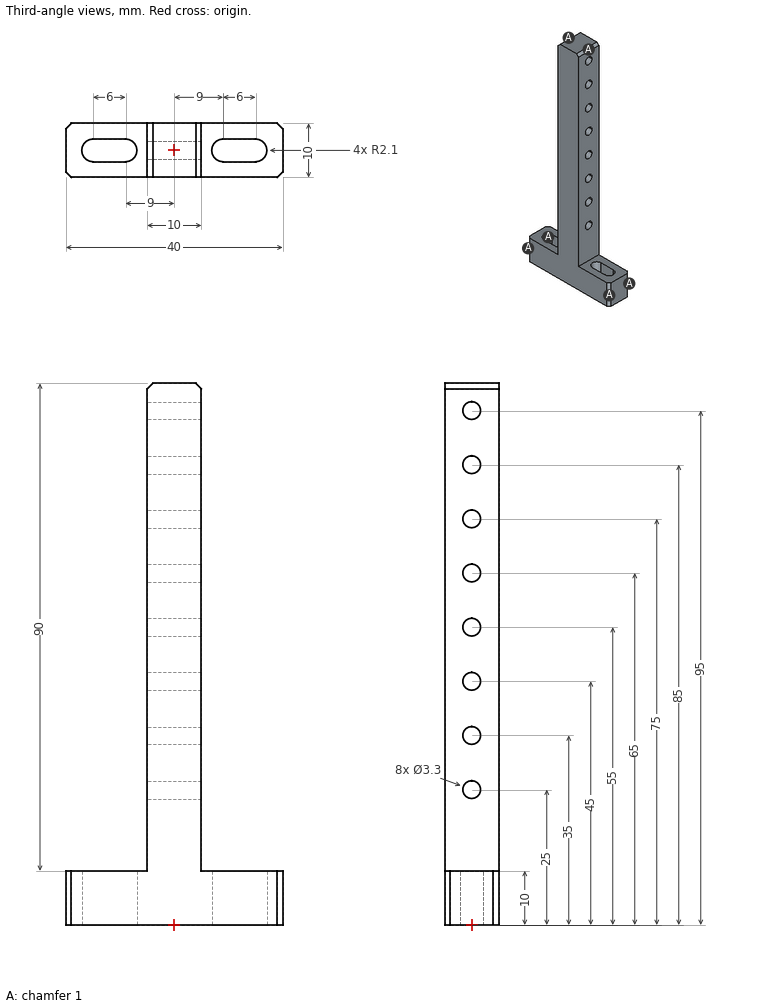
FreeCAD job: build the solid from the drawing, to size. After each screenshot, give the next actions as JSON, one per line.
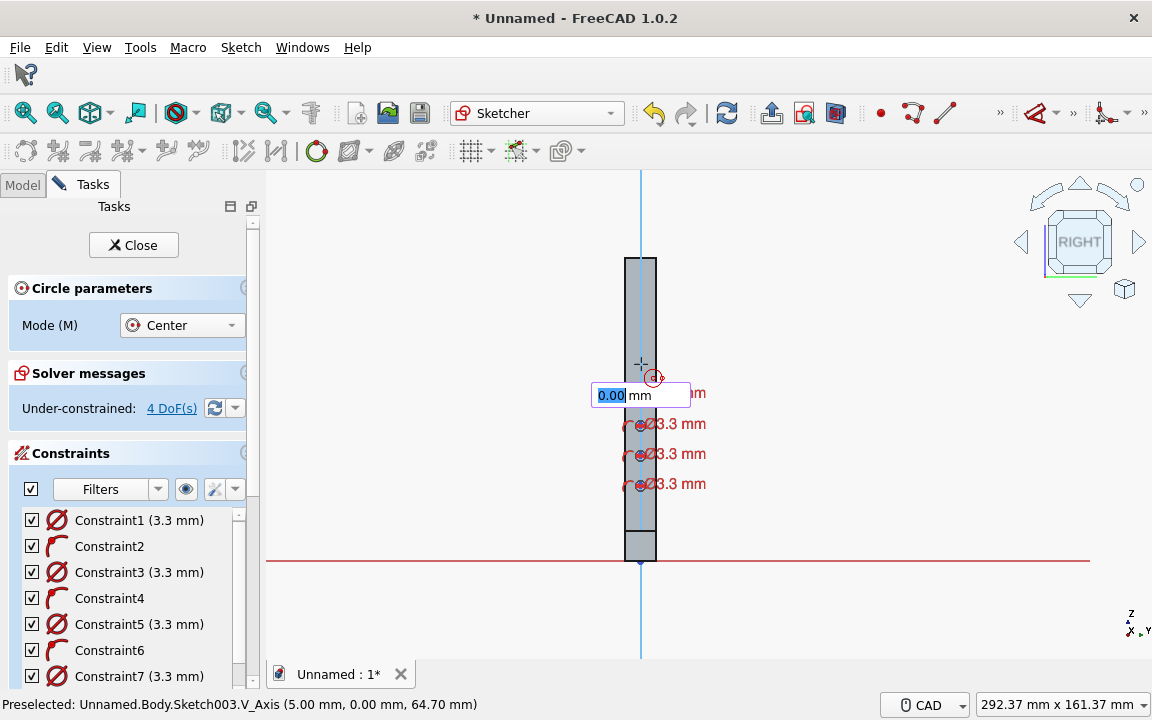
{"action": "scroll", "coordinate": [645, 362], "scroll_direction": "up", "scroll_amount": 7}
{"action": "mouse_move", "coordinate": [645, 362]}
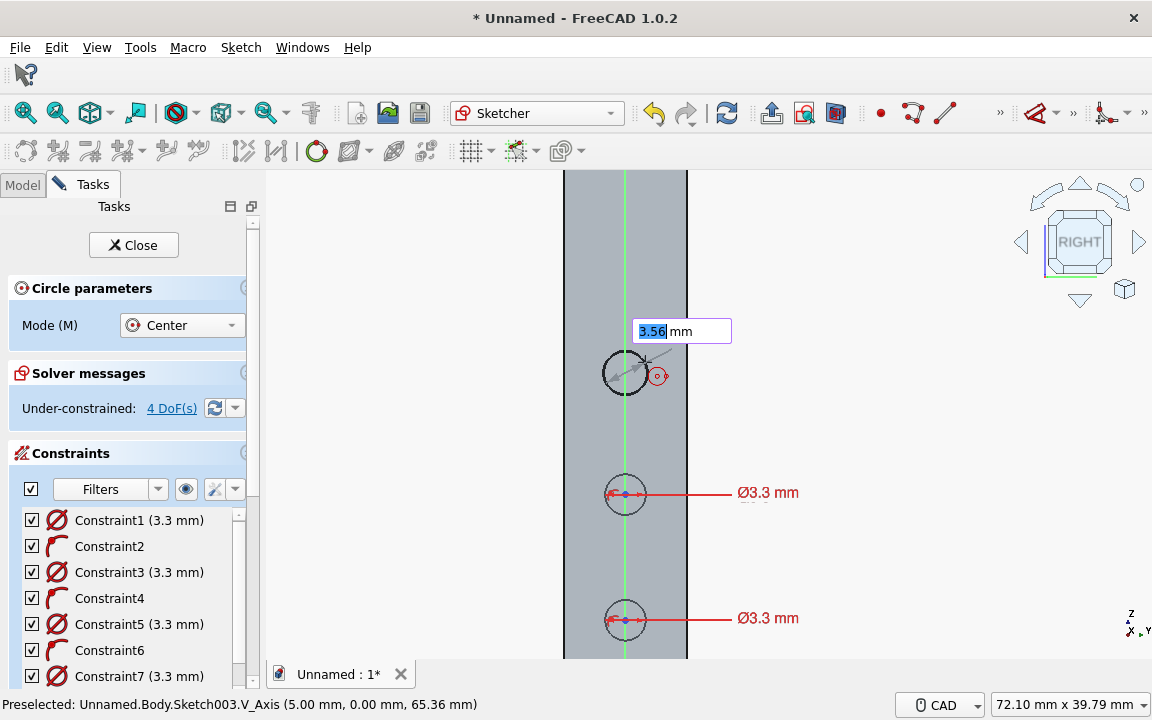
{"action": "type", "text": "3.3"}
{"action": "key", "text": "Return"}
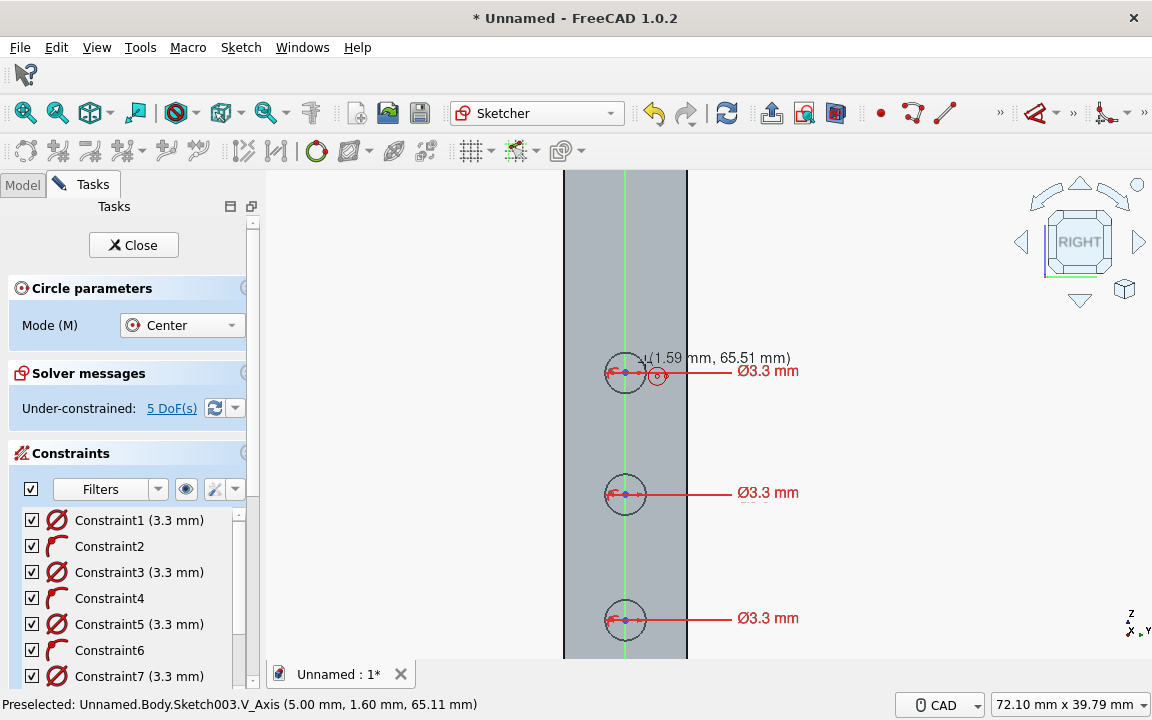
{"action": "scroll", "coordinate": [645, 362], "scroll_direction": "down", "scroll_amount": 7}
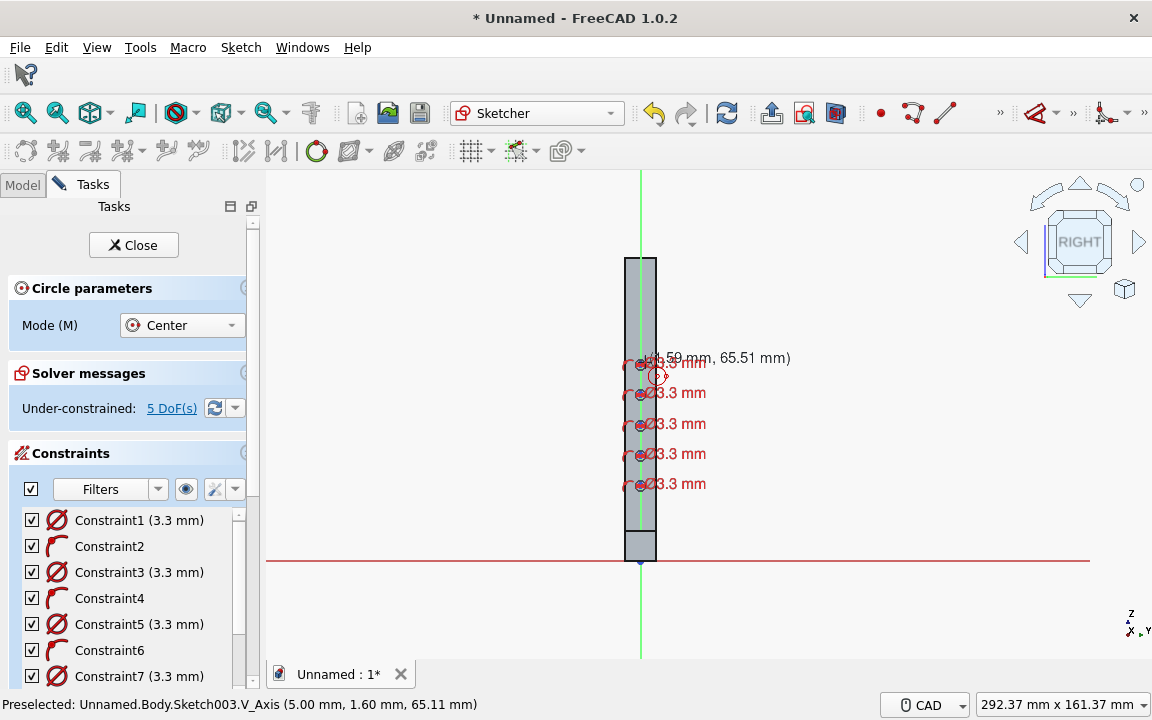
{"action": "left_click", "coordinate": [641, 334]}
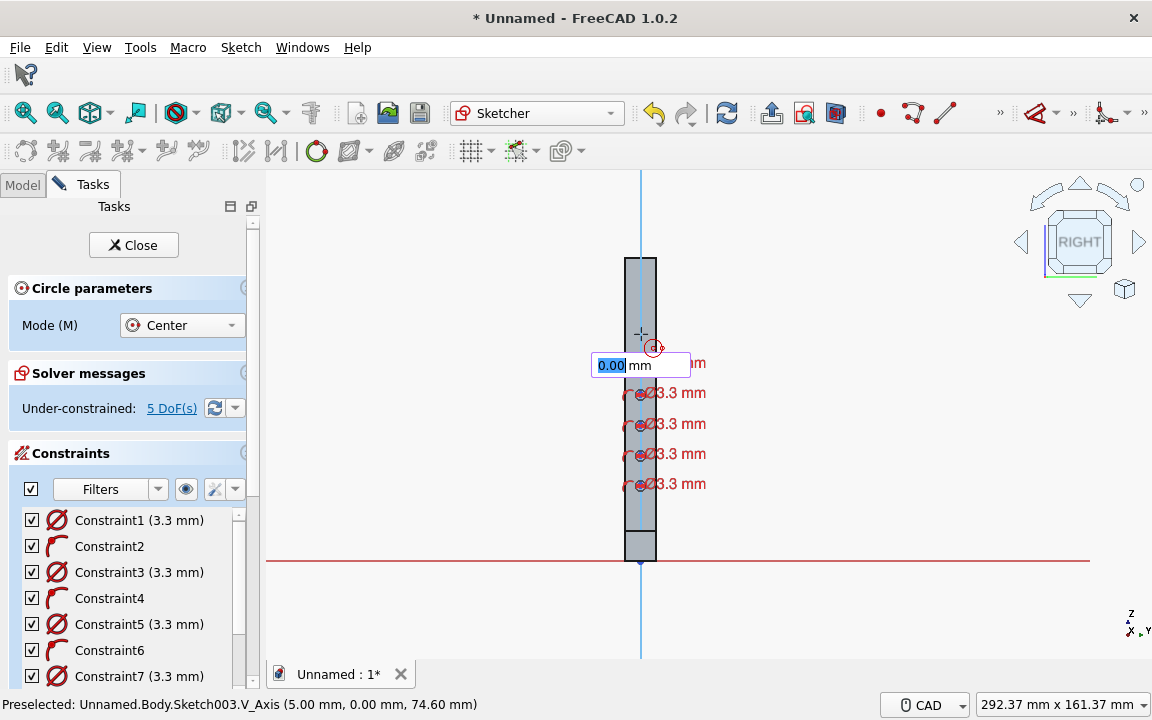
{"action": "scroll", "coordinate": [645, 332], "scroll_direction": "up", "scroll_amount": 7}
{"action": "mouse_move", "coordinate": [645, 331]}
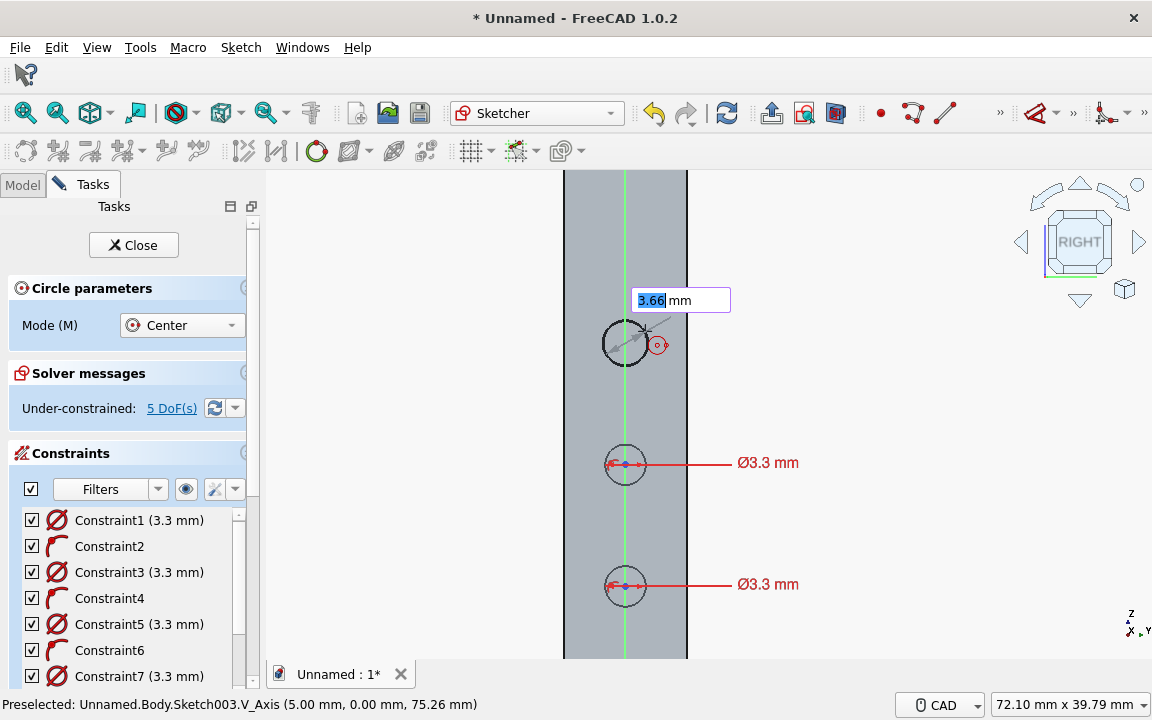
{"action": "type", "text": "3.3"}
{"action": "key", "text": "Return"}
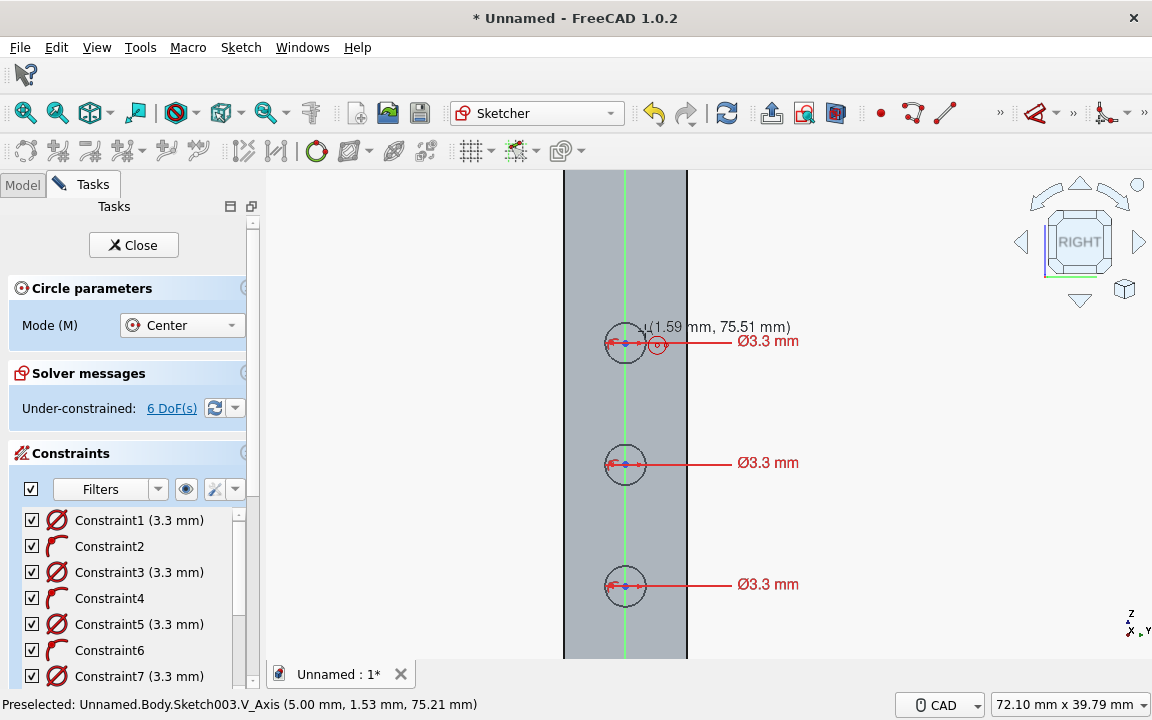
{"action": "scroll", "coordinate": [645, 332], "scroll_direction": "down", "scroll_amount": 7}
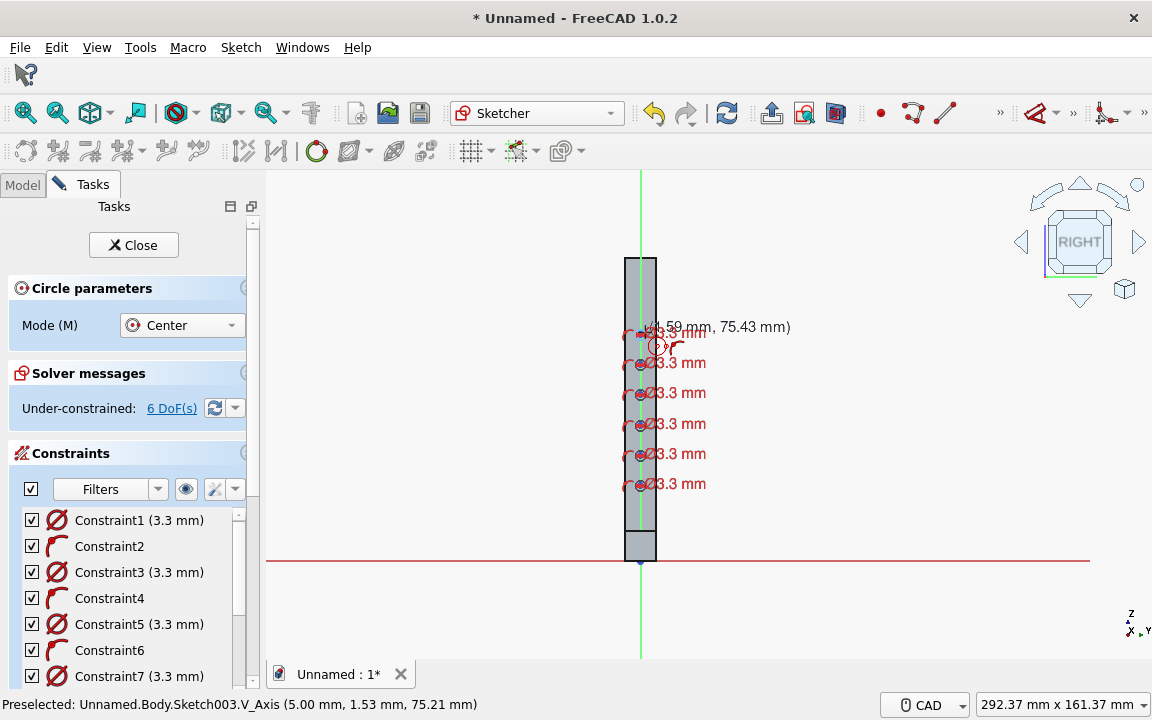
{"action": "left_click", "coordinate": [641, 303]}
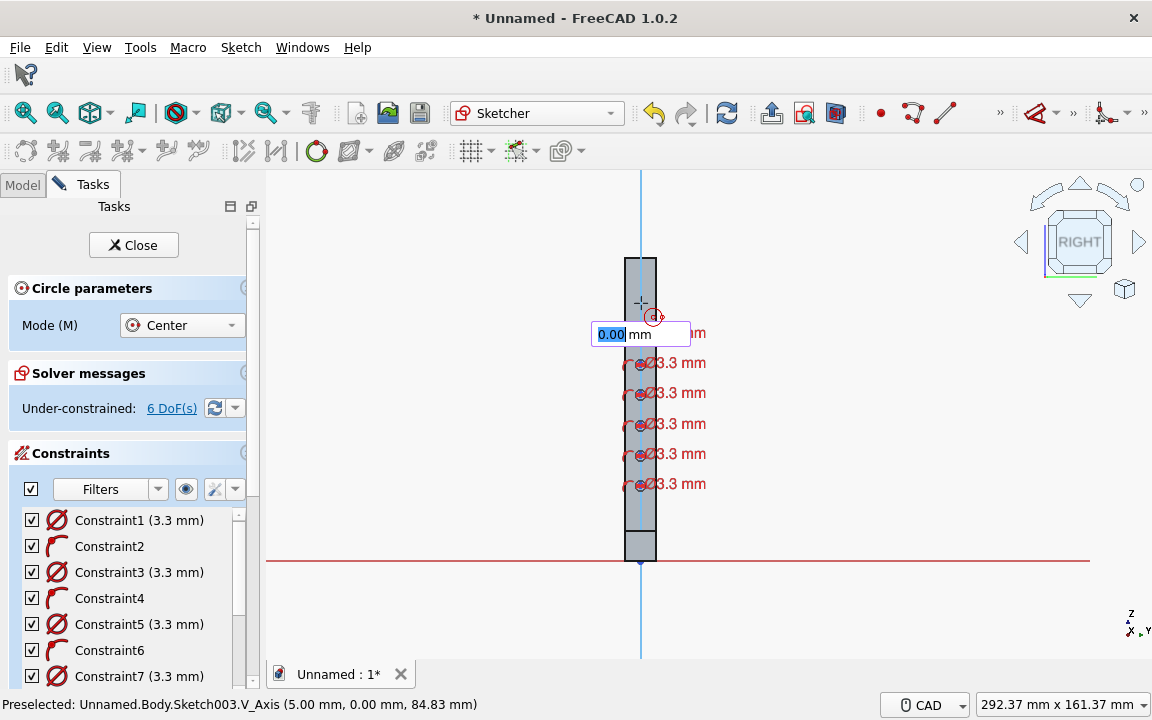
{"action": "scroll", "coordinate": [645, 302], "scroll_direction": "up", "scroll_amount": 7}
{"action": "mouse_move", "coordinate": [645, 300]}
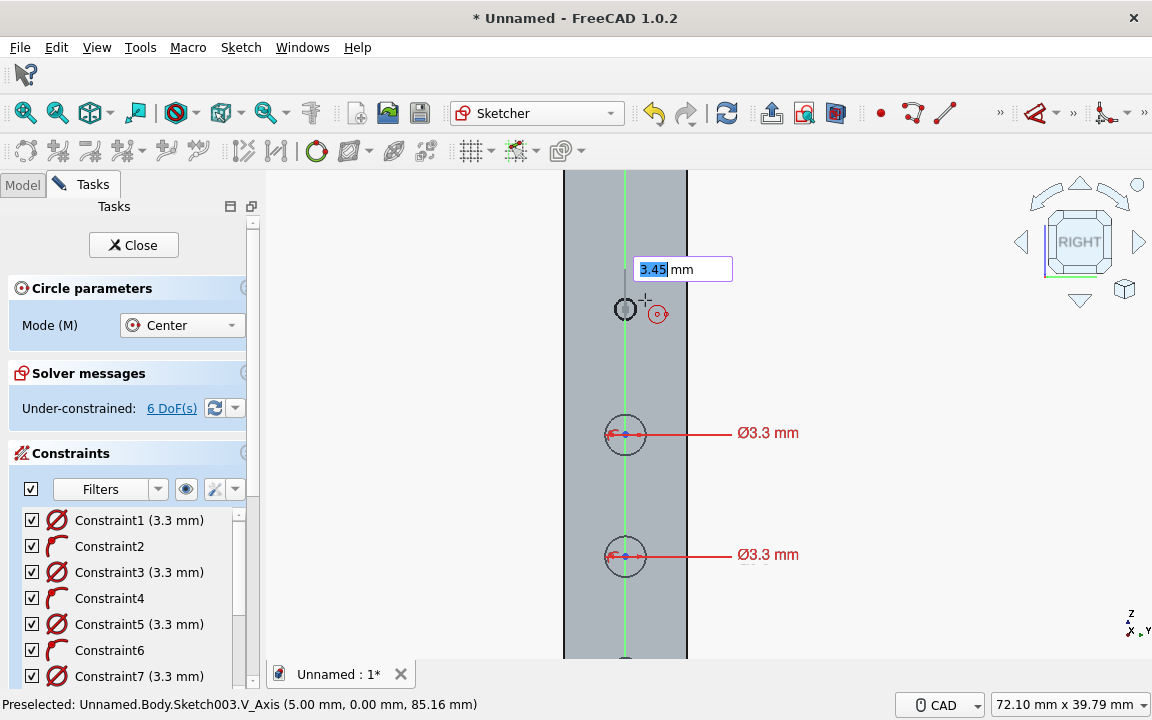
{"action": "type", "text": "3.3"}
{"action": "key", "text": "Return"}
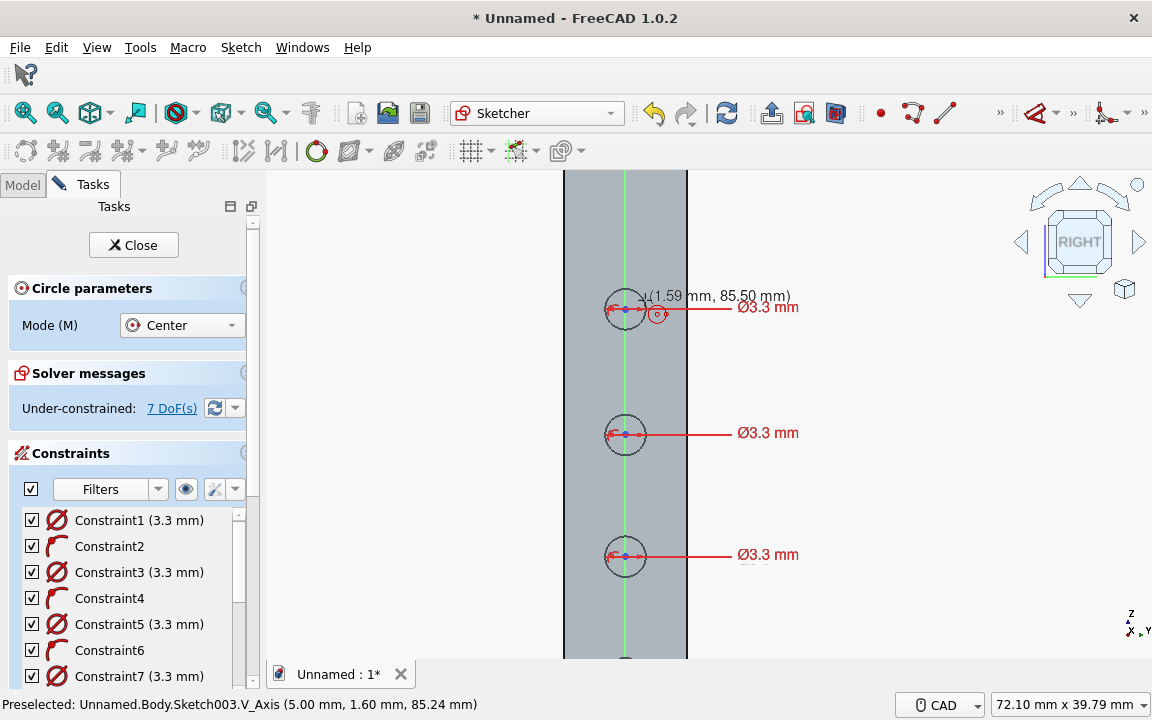
{"action": "scroll", "coordinate": [645, 302], "scroll_direction": "down", "scroll_amount": 7}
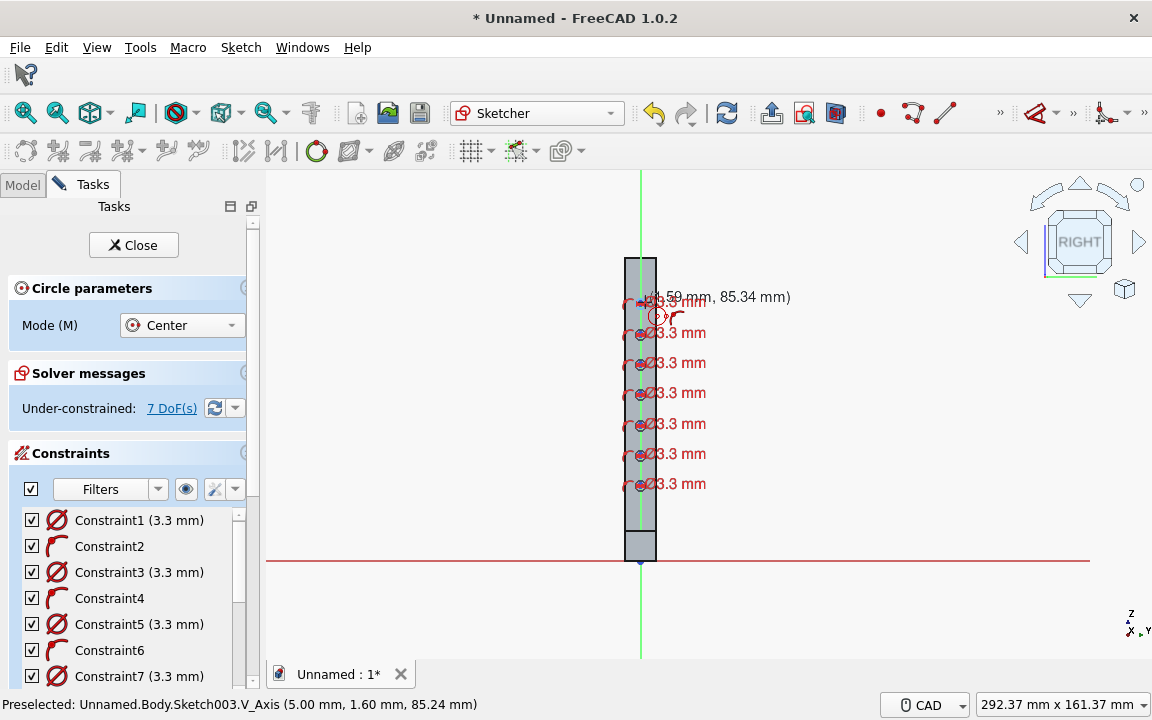
{"action": "scroll", "coordinate": [641, 273], "scroll_direction": "up", "scroll_amount": 8}